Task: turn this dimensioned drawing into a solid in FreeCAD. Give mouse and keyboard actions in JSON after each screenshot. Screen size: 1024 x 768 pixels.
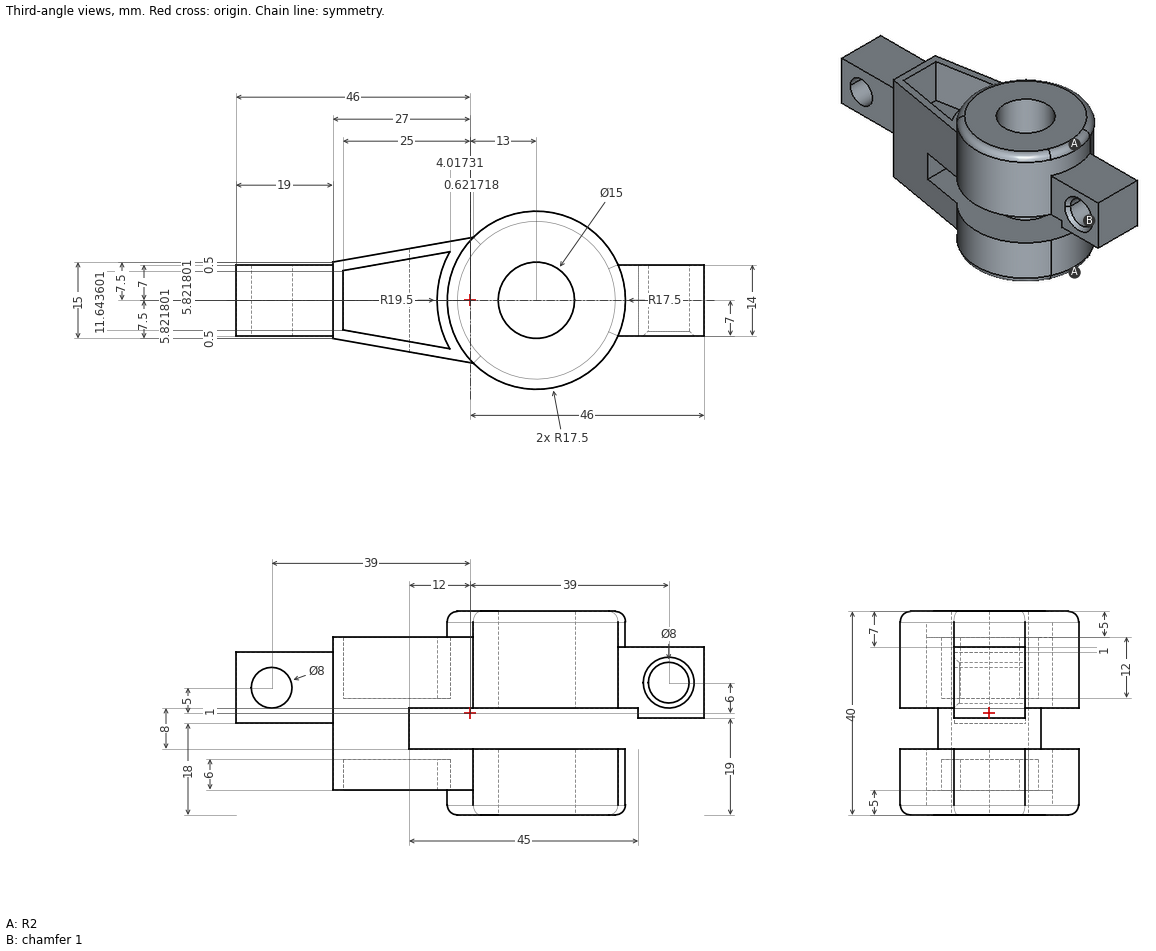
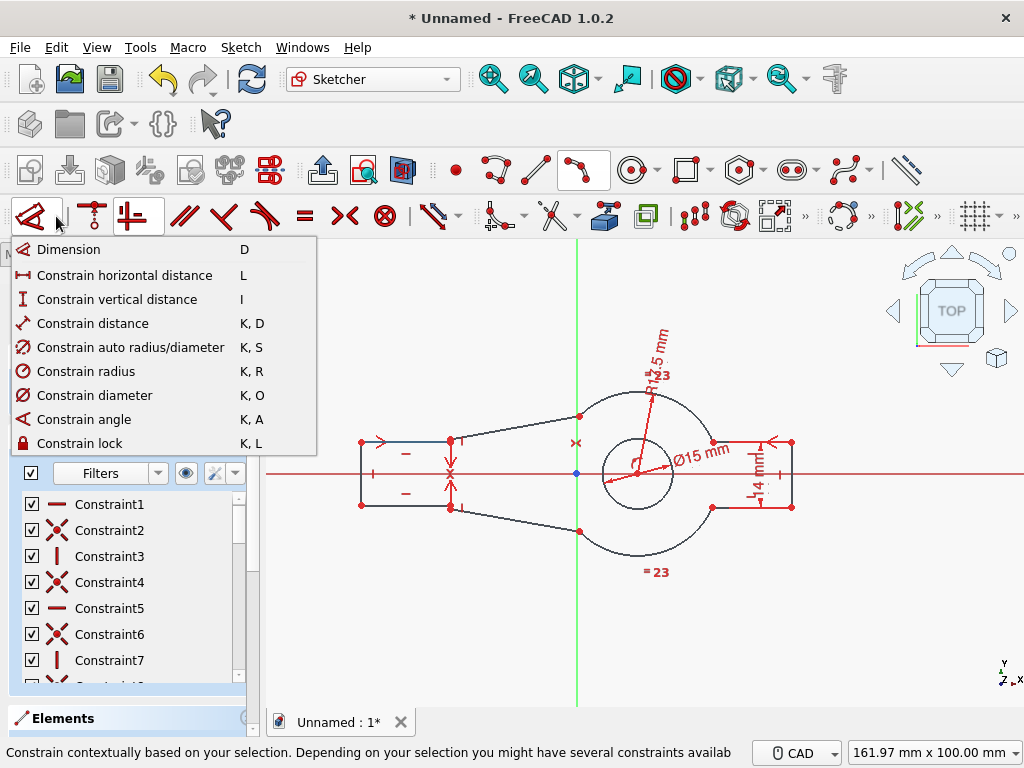
{"action": "left_click", "coordinate": [164, 275]}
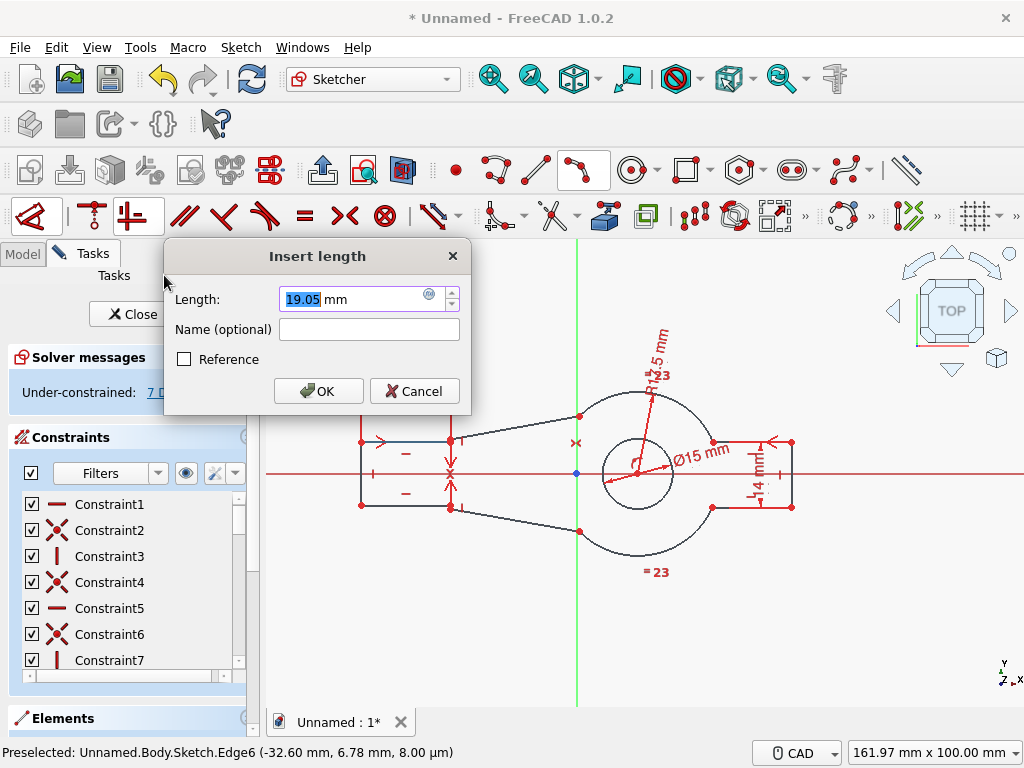
{"action": "type", "text": "19"}
{"action": "key", "text": "Return"}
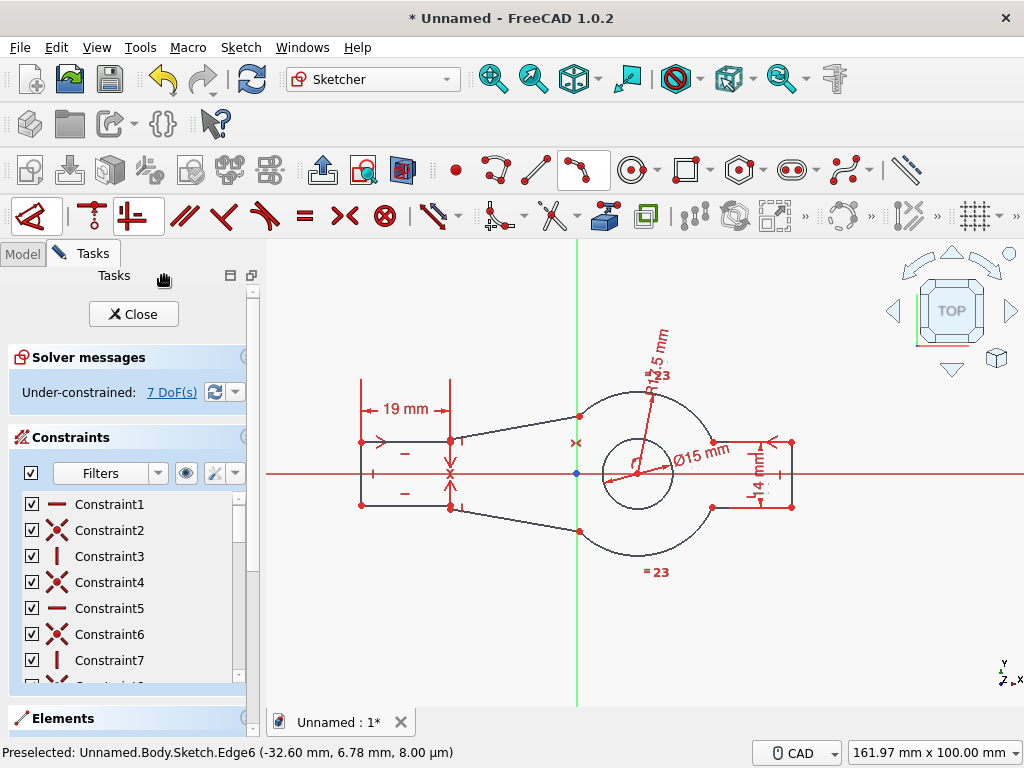
{"action": "left_click", "coordinate": [361, 461]}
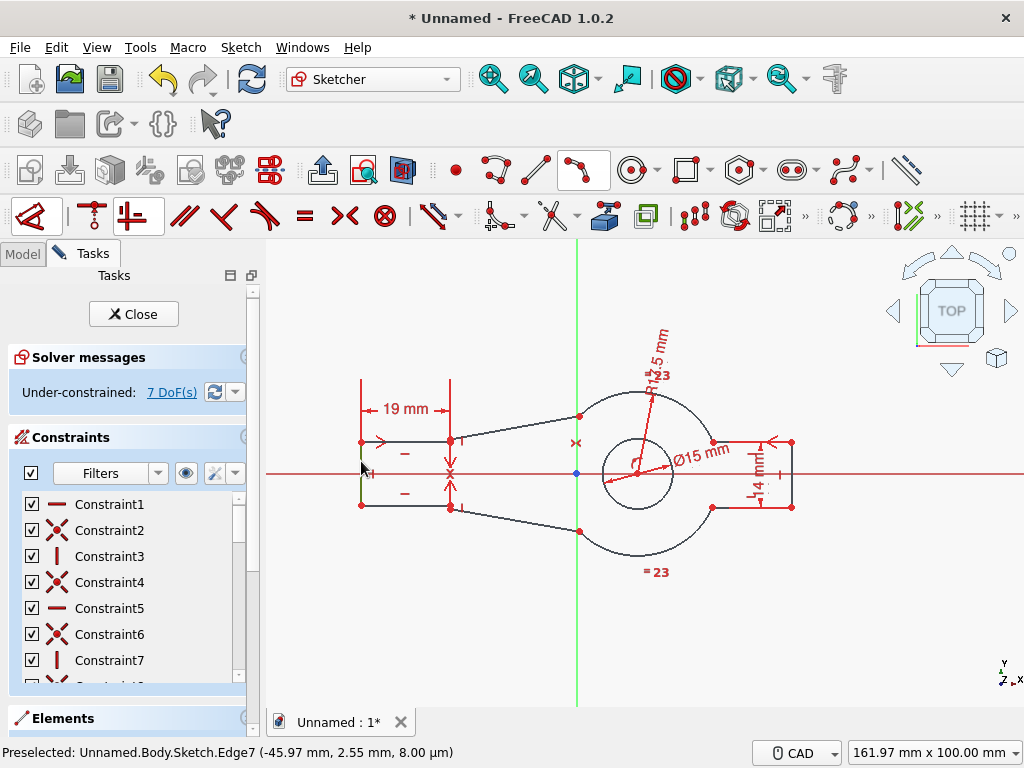
{"action": "key", "text": "i"}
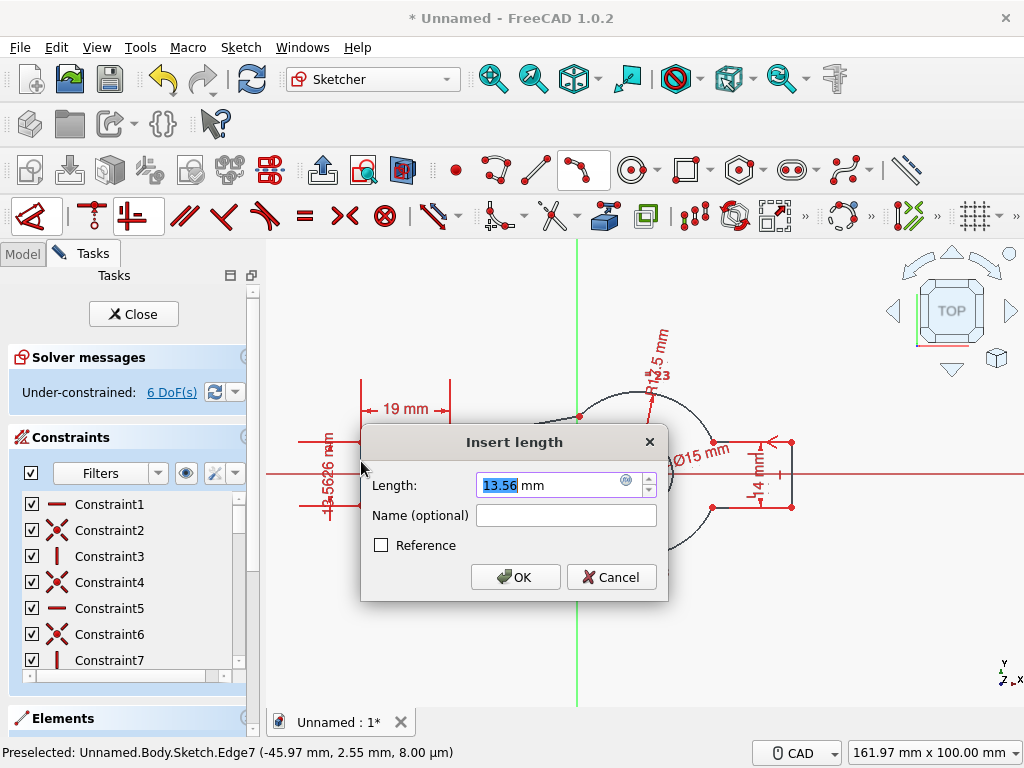
{"action": "type", "text": "14"}
{"action": "key", "text": "Return"}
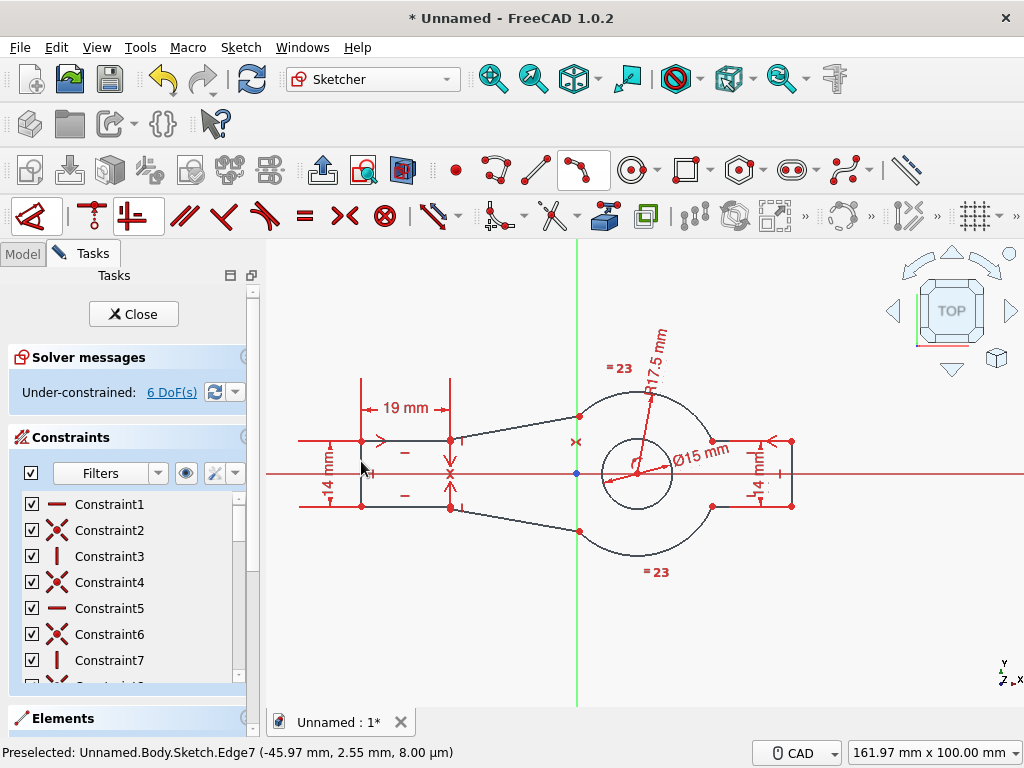
{"action": "left_click", "coordinate": [637, 474]}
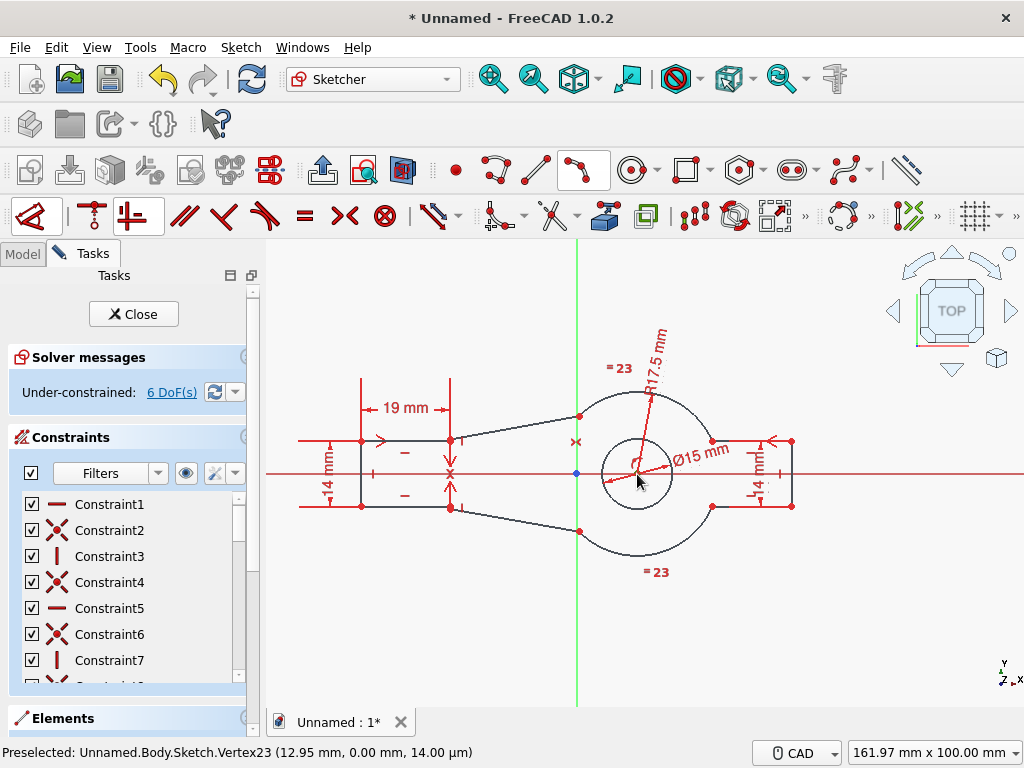
{"action": "left_click", "coordinate": [56, 216]}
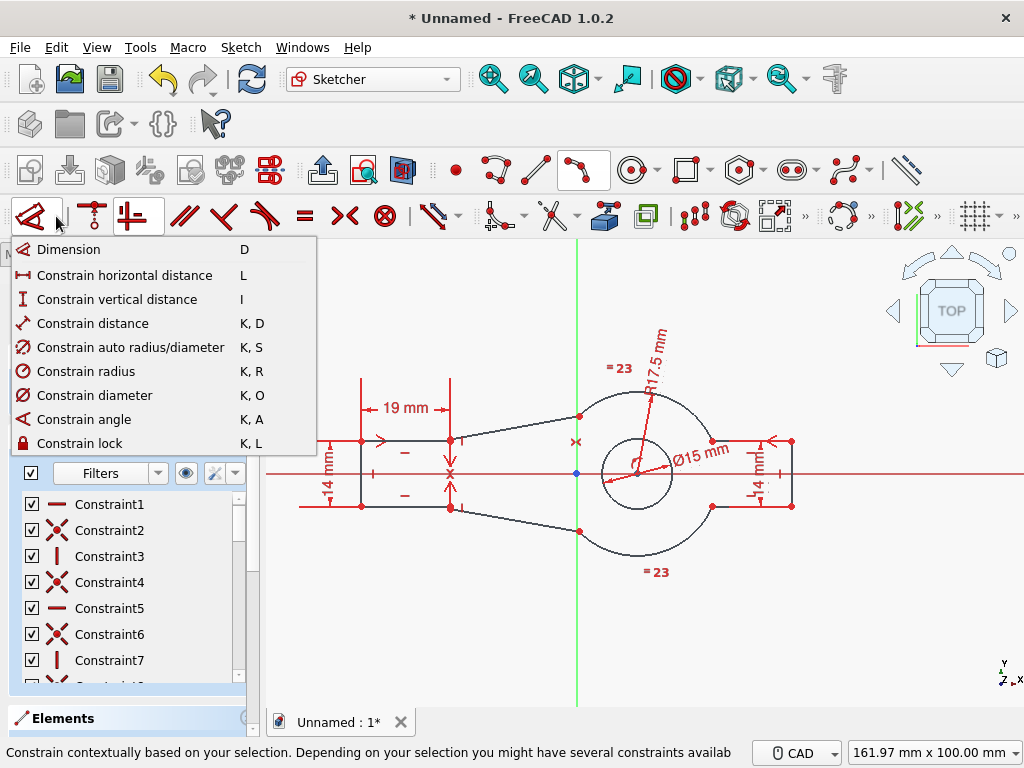
{"action": "left_click", "coordinate": [164, 275]}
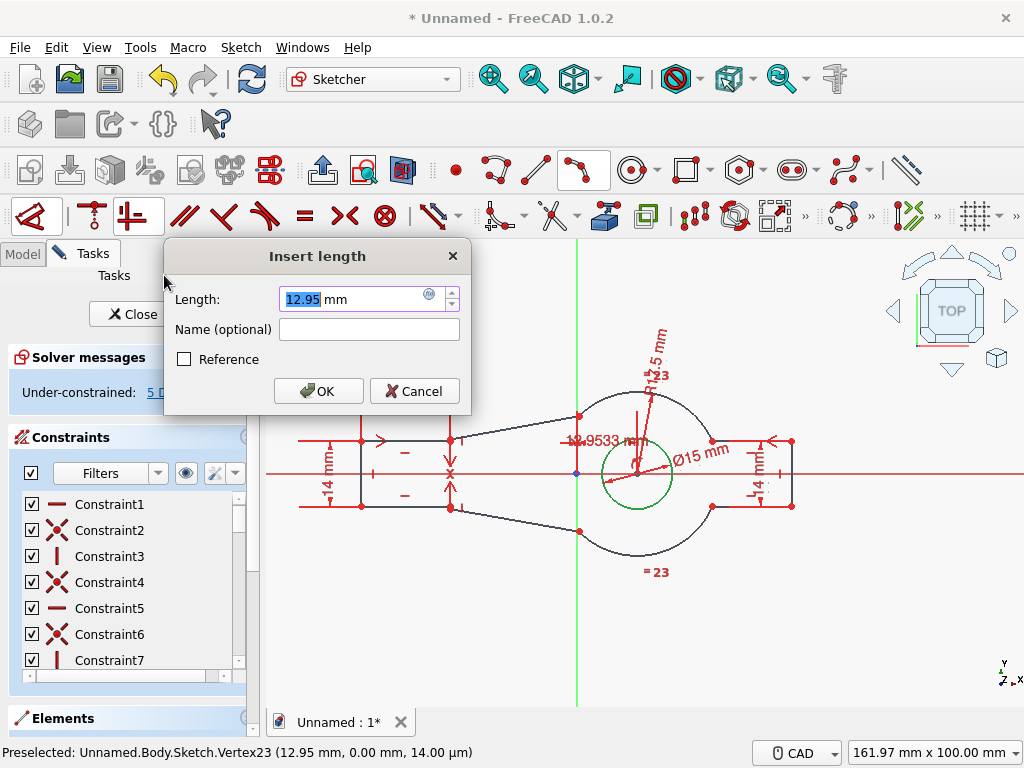
{"action": "type", "text": "13"}
{"action": "key", "text": "Return"}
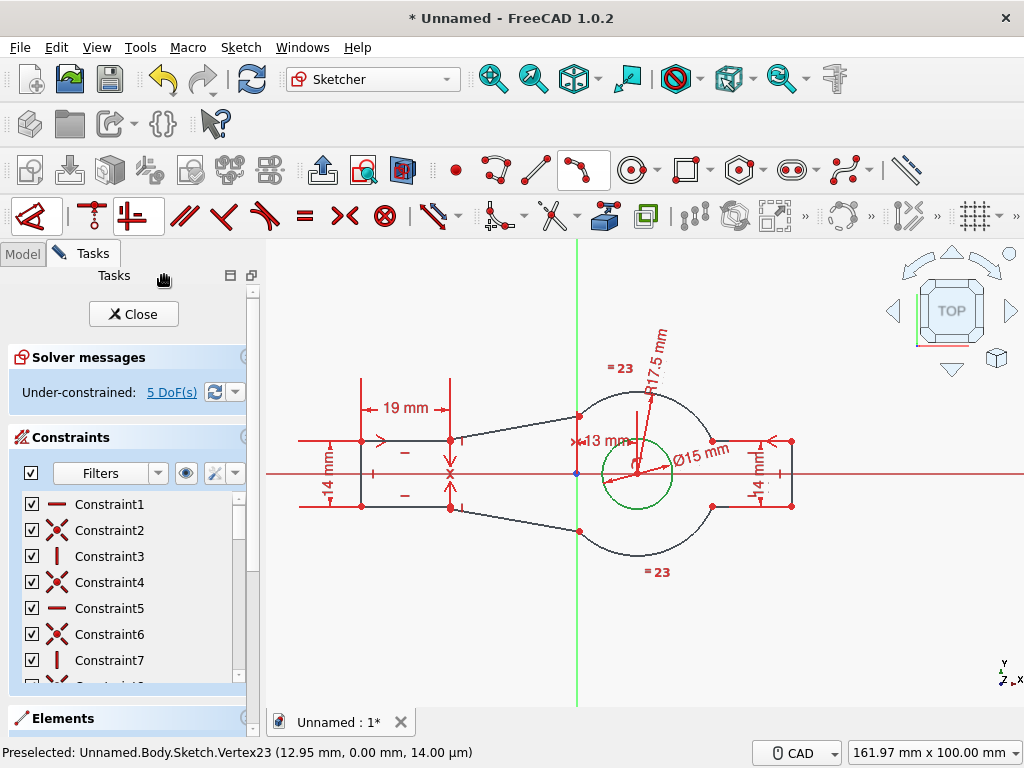
{"action": "scroll", "coordinate": [450, 440], "scroll_direction": "up", "scroll_amount": 15}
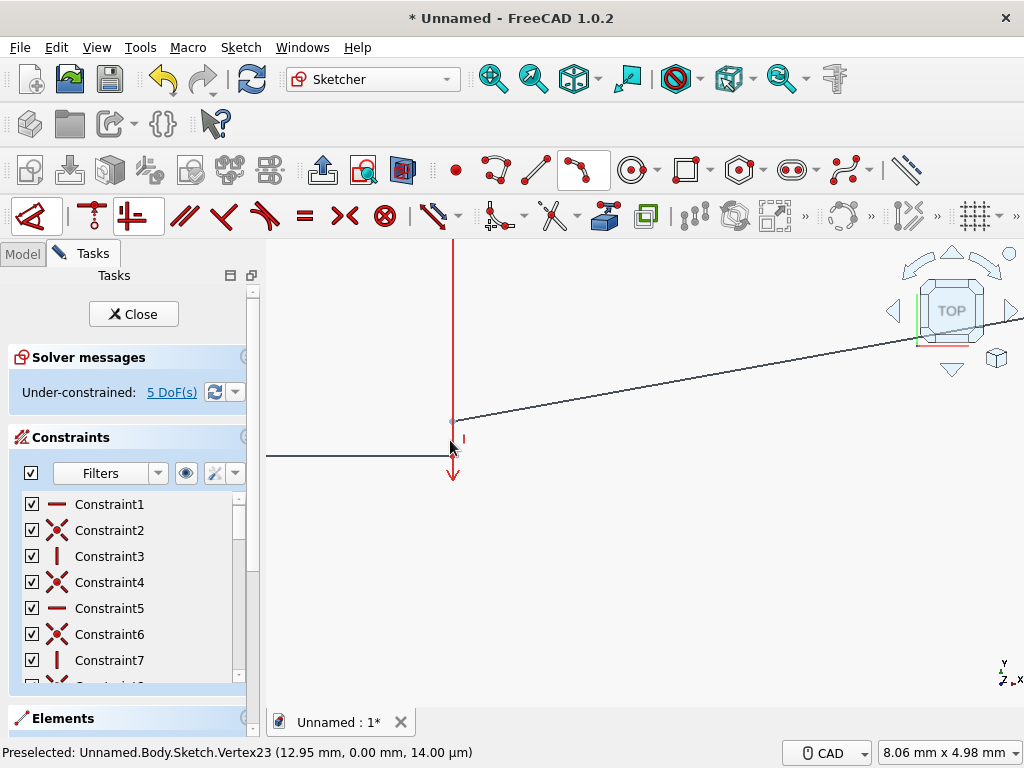
{"action": "left_click", "coordinate": [453, 439]}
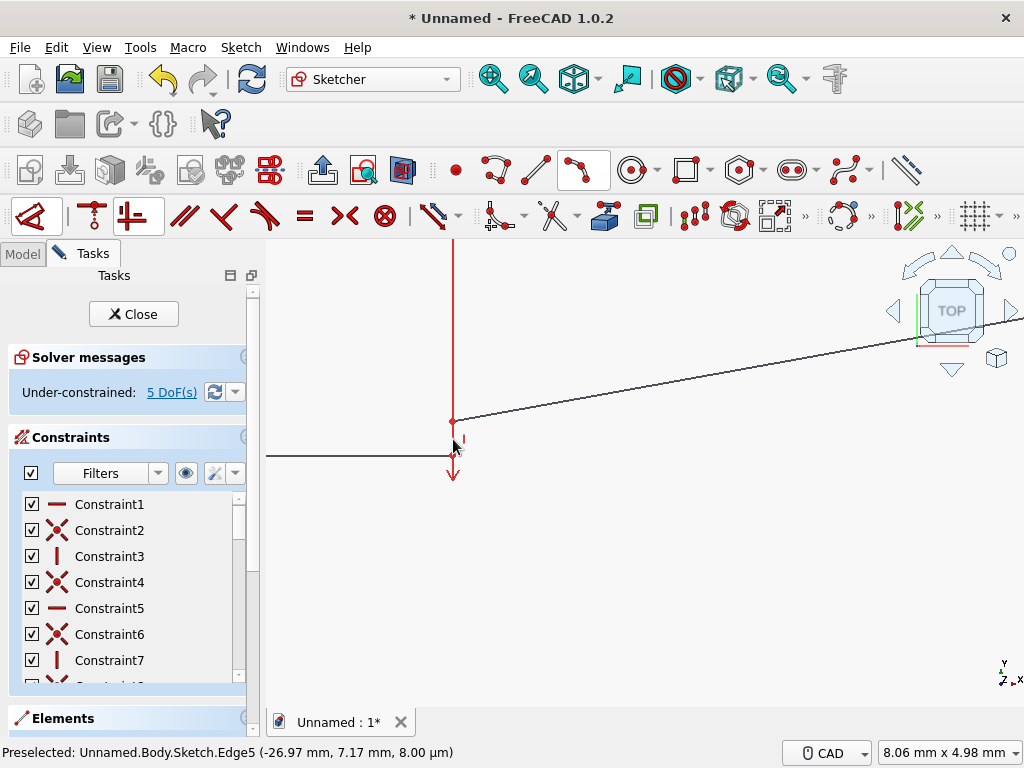
{"action": "key", "text": "i"}